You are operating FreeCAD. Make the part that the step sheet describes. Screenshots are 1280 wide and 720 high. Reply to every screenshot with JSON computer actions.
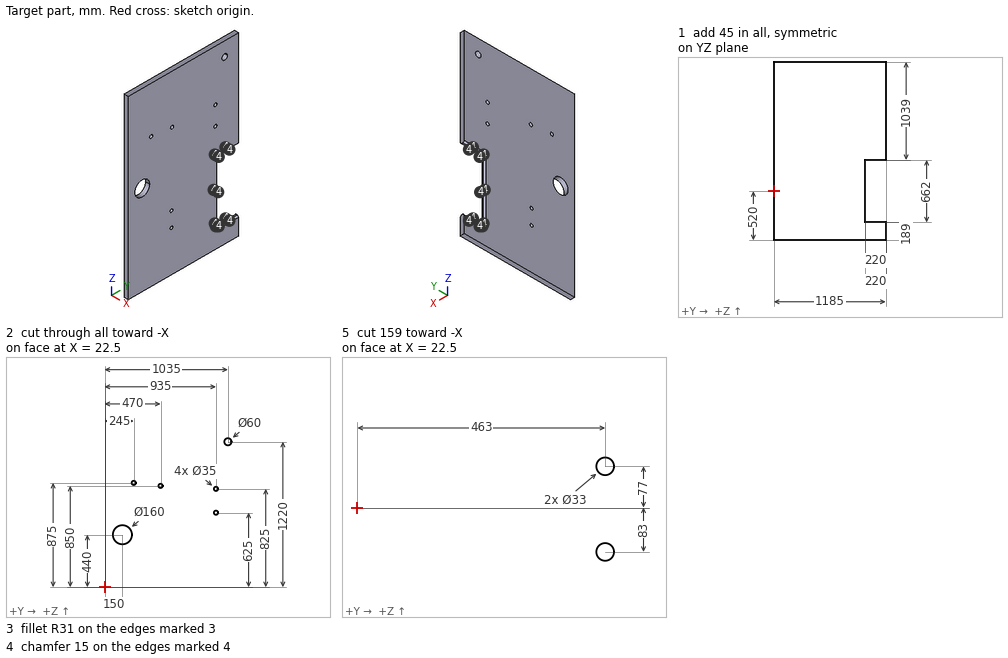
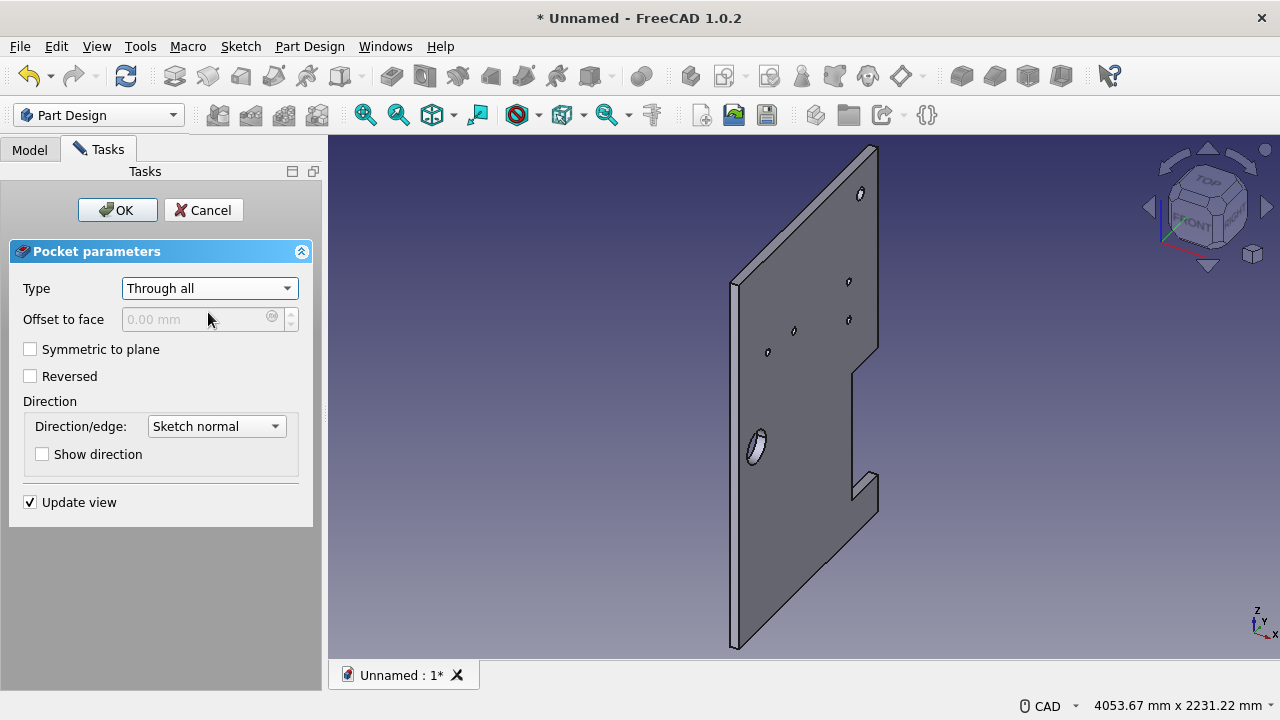
{"action": "left_click", "coordinate": [118, 210]}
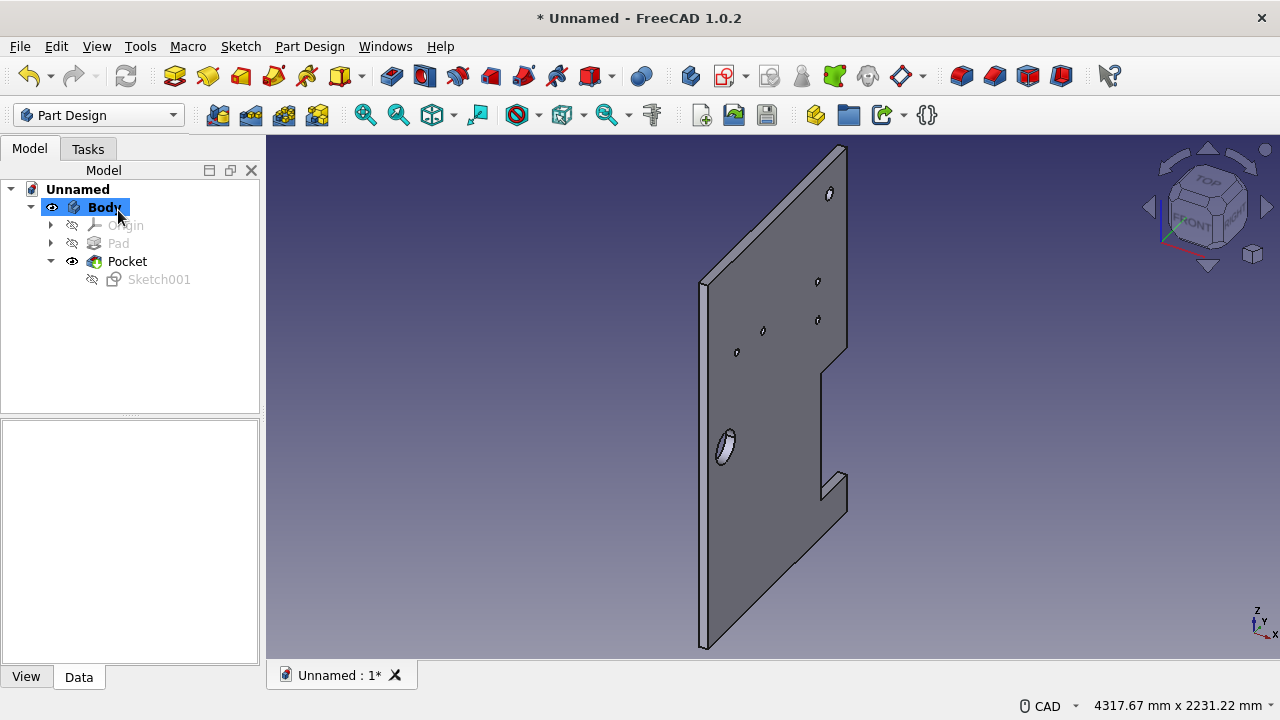
{"action": "scroll", "coordinate": [817, 371], "scroll_direction": "up", "scroll_amount": 7}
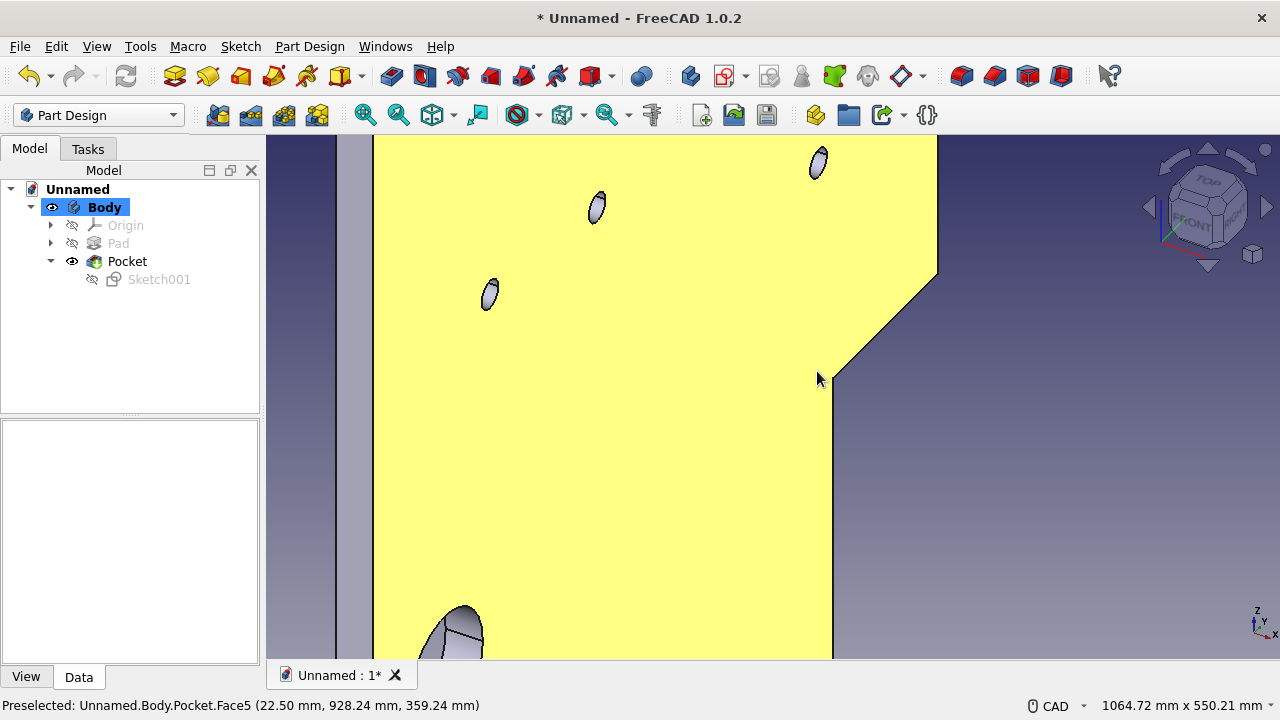
{"action": "left_click", "coordinate": [366, 116]}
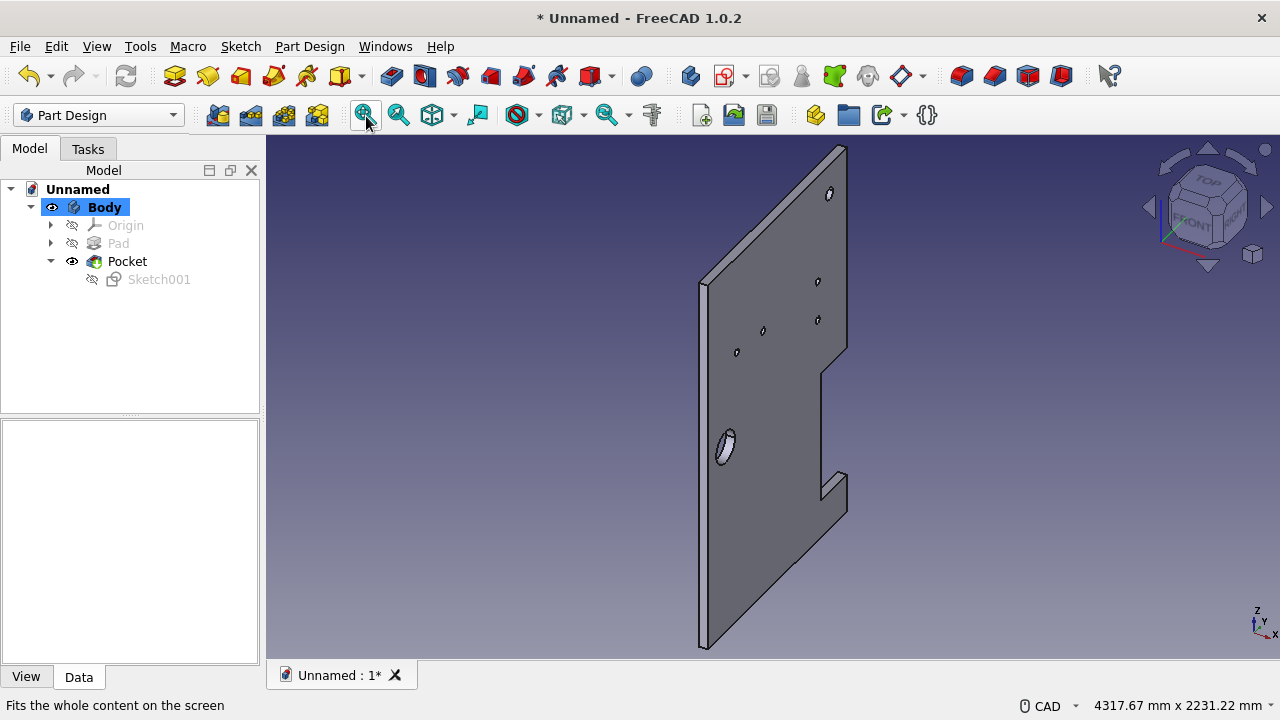
{"action": "key", "text": "0"}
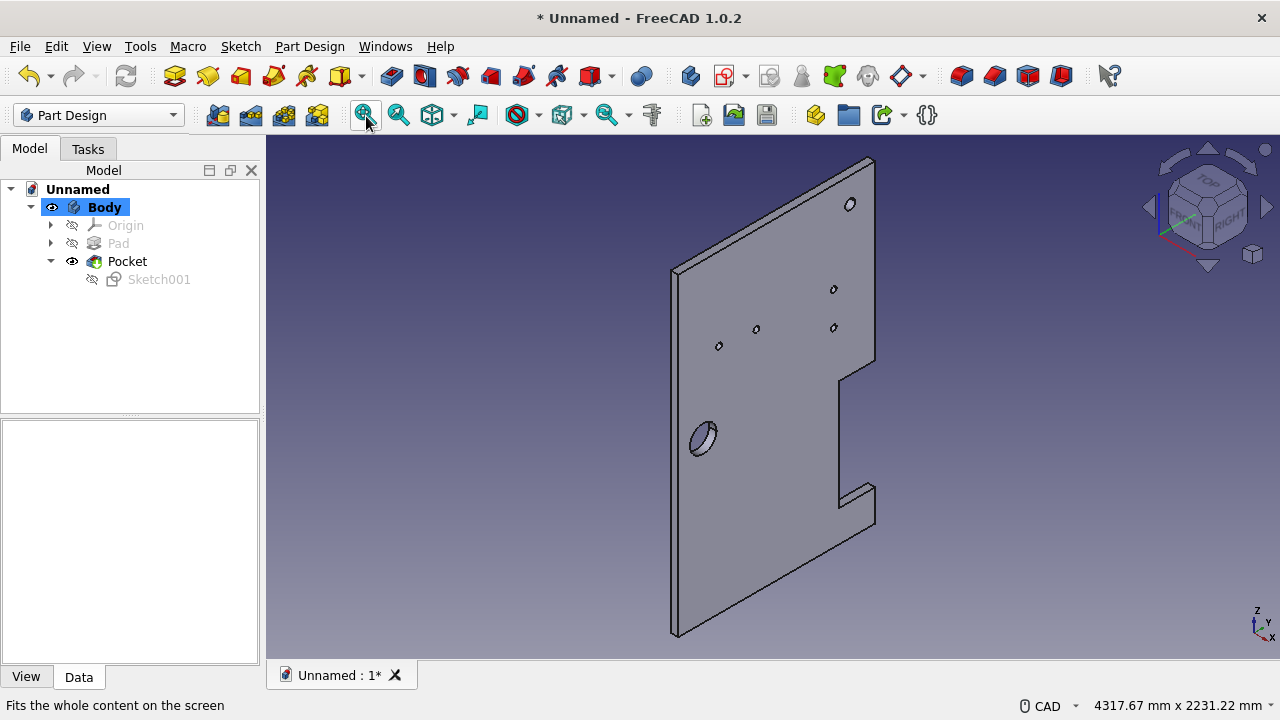
{"action": "scroll", "coordinate": [835, 378], "scroll_direction": "up", "scroll_amount": 7}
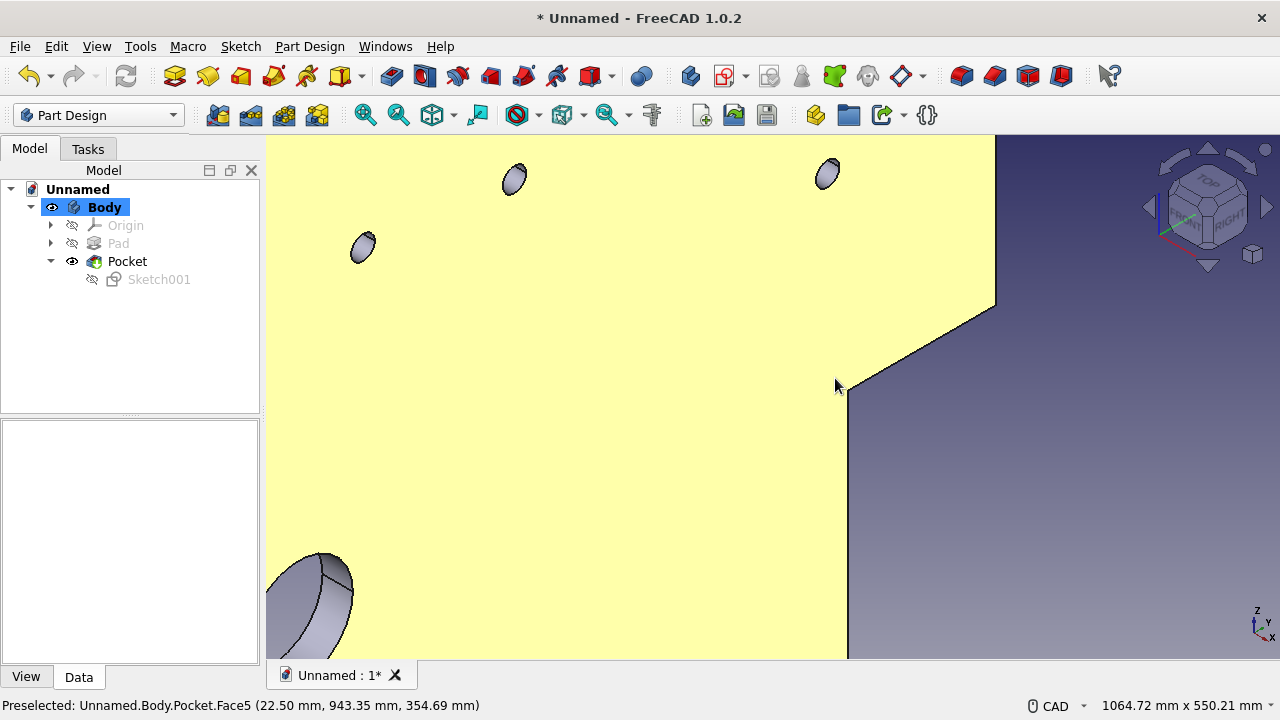
{"action": "left_click", "coordinate": [366, 116]}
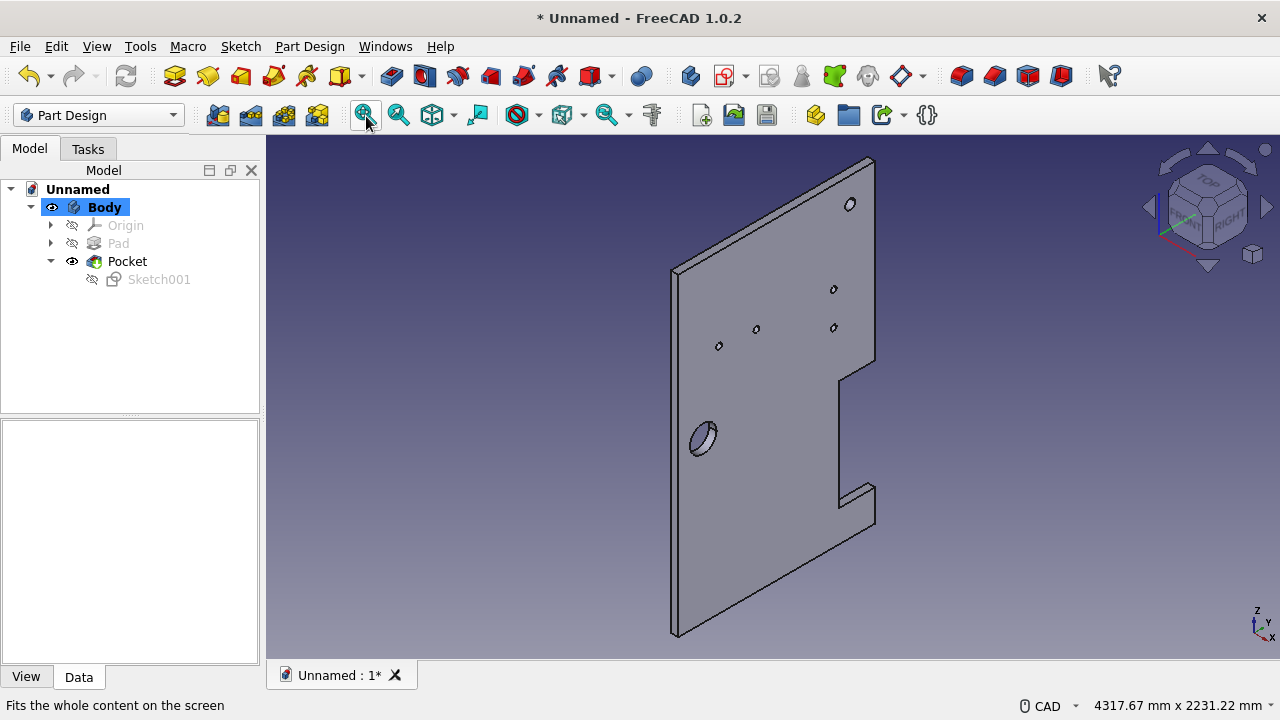
{"action": "key", "text": "2"}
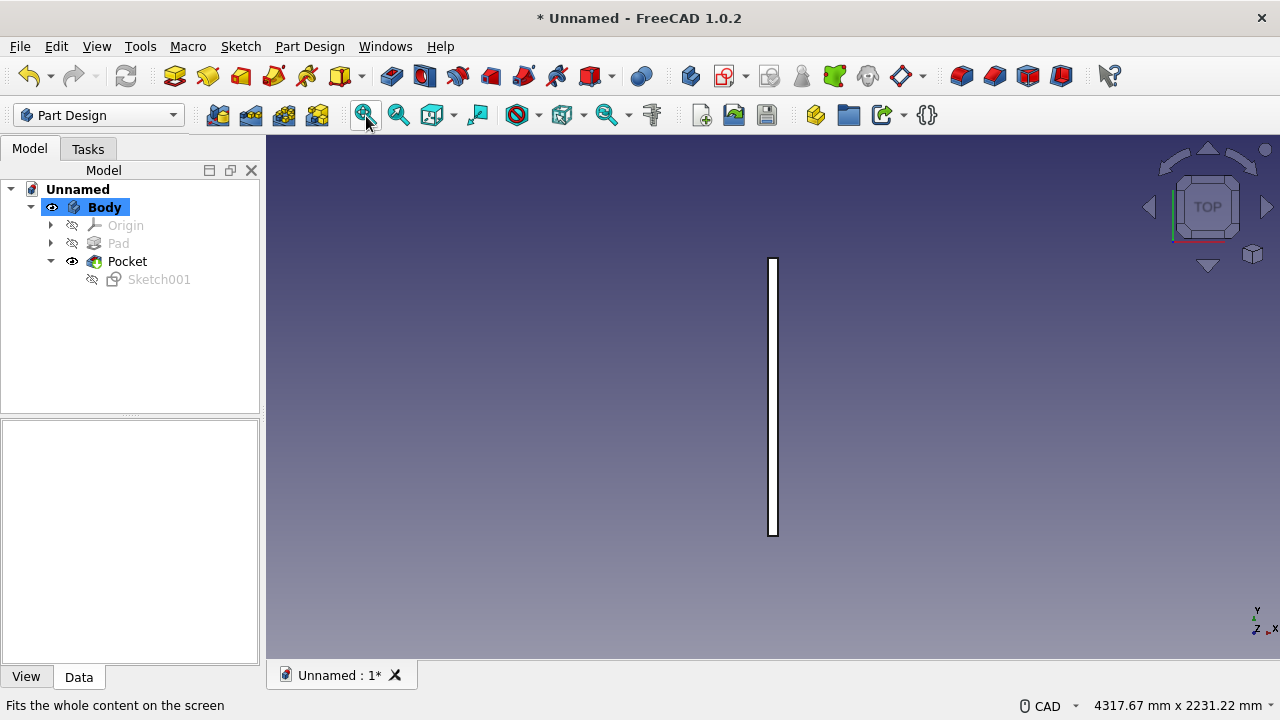
{"action": "scroll", "coordinate": [773, 309], "scroll_direction": "up", "scroll_amount": 7}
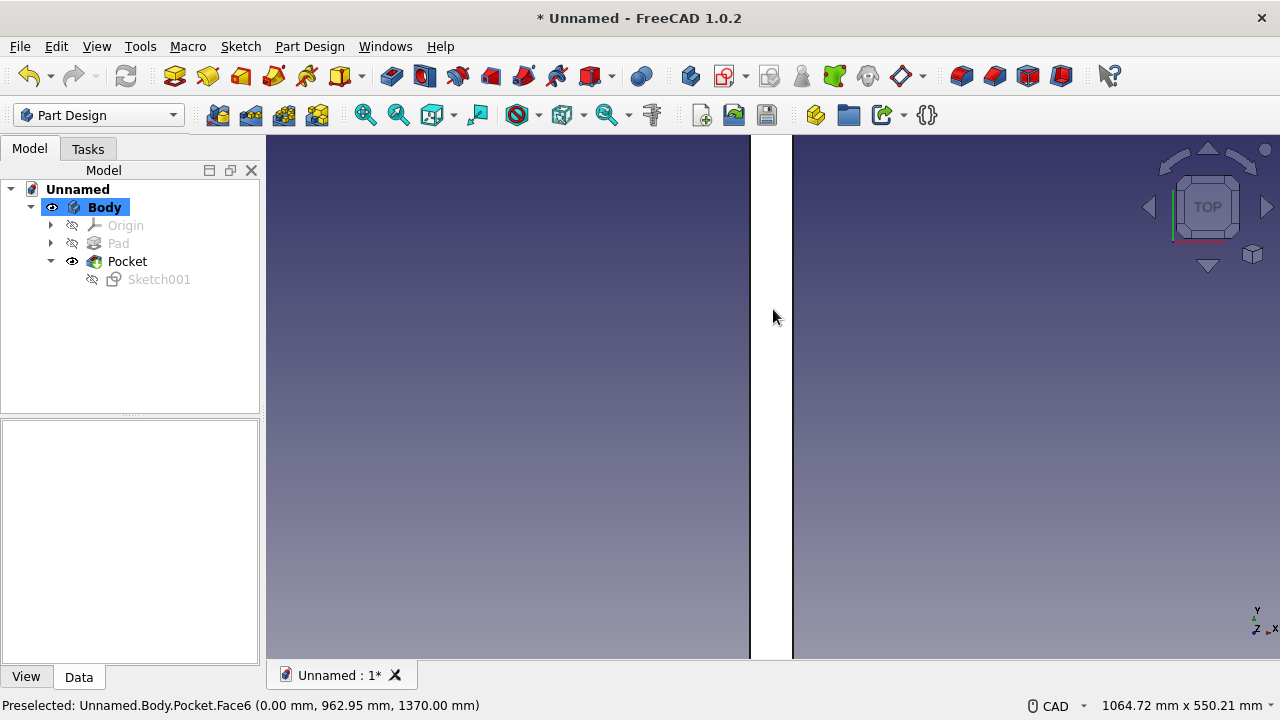
{"action": "left_click", "coordinate": [366, 116]}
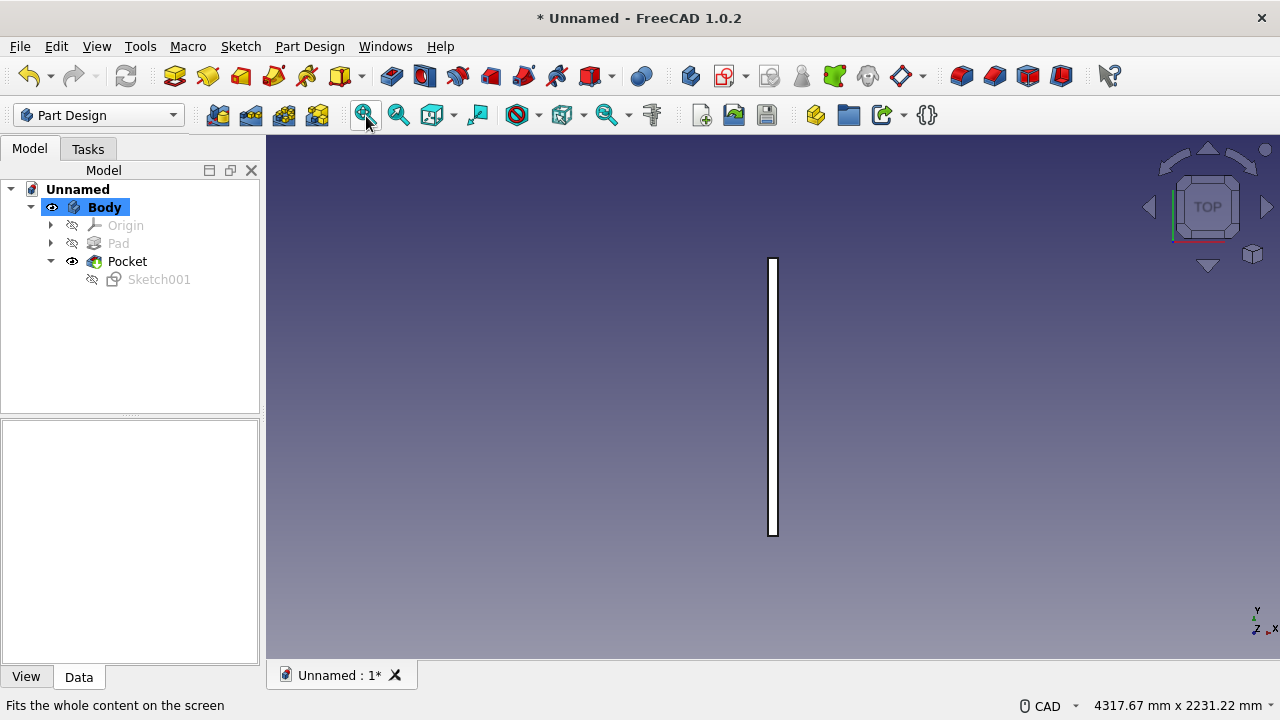
{"action": "key", "text": "1"}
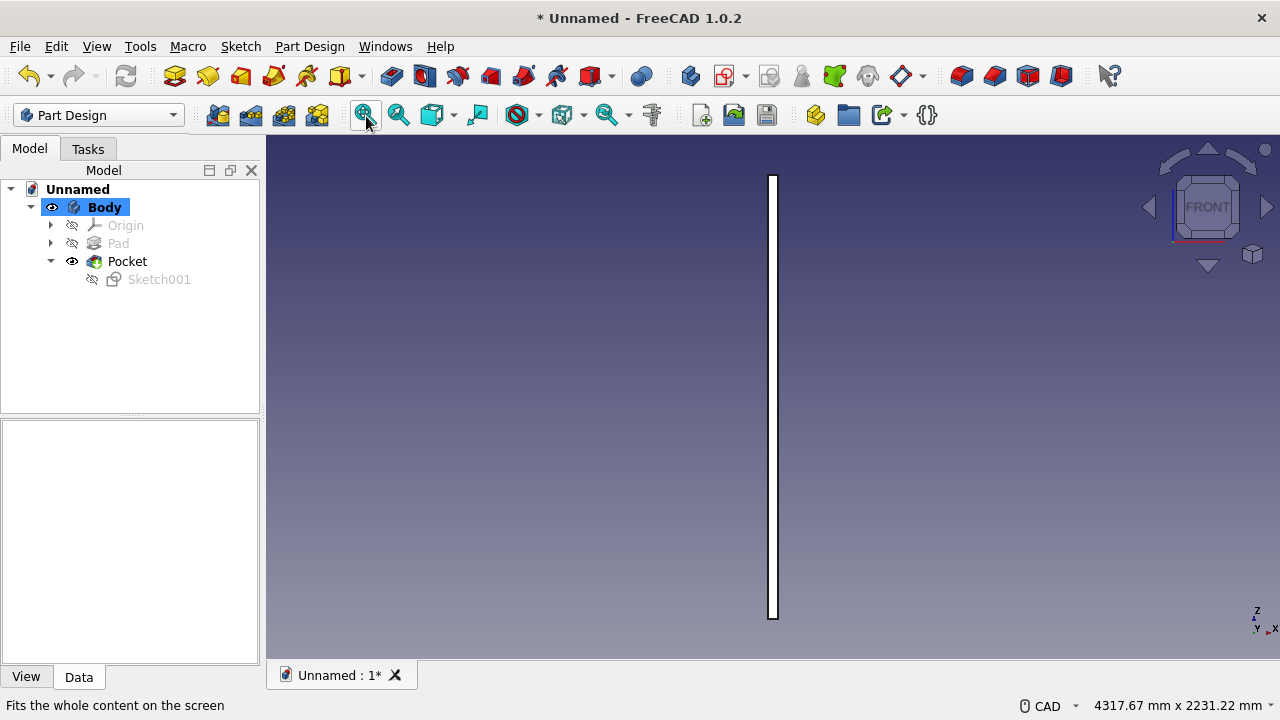
{"action": "scroll", "coordinate": [773, 418], "scroll_direction": "up", "scroll_amount": 7}